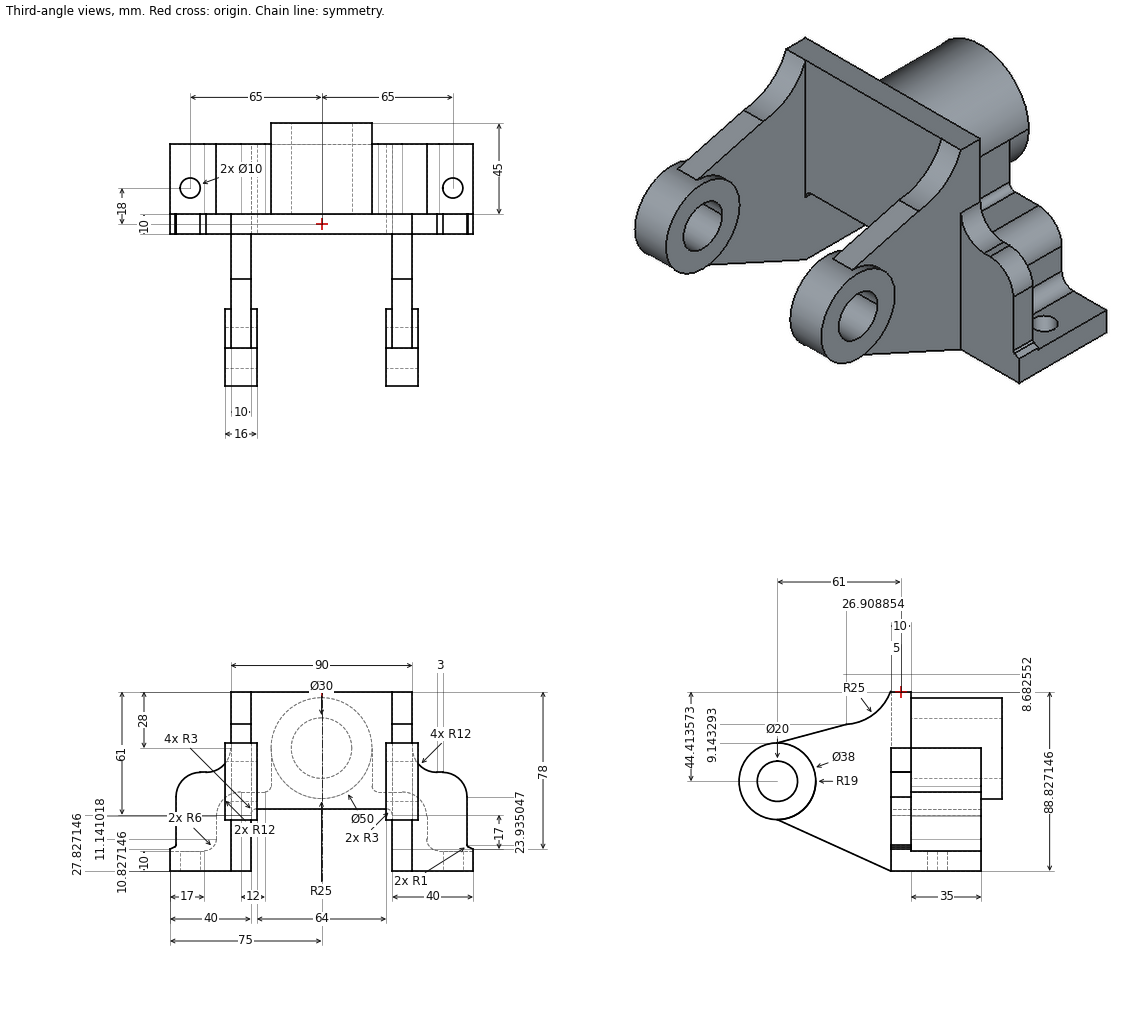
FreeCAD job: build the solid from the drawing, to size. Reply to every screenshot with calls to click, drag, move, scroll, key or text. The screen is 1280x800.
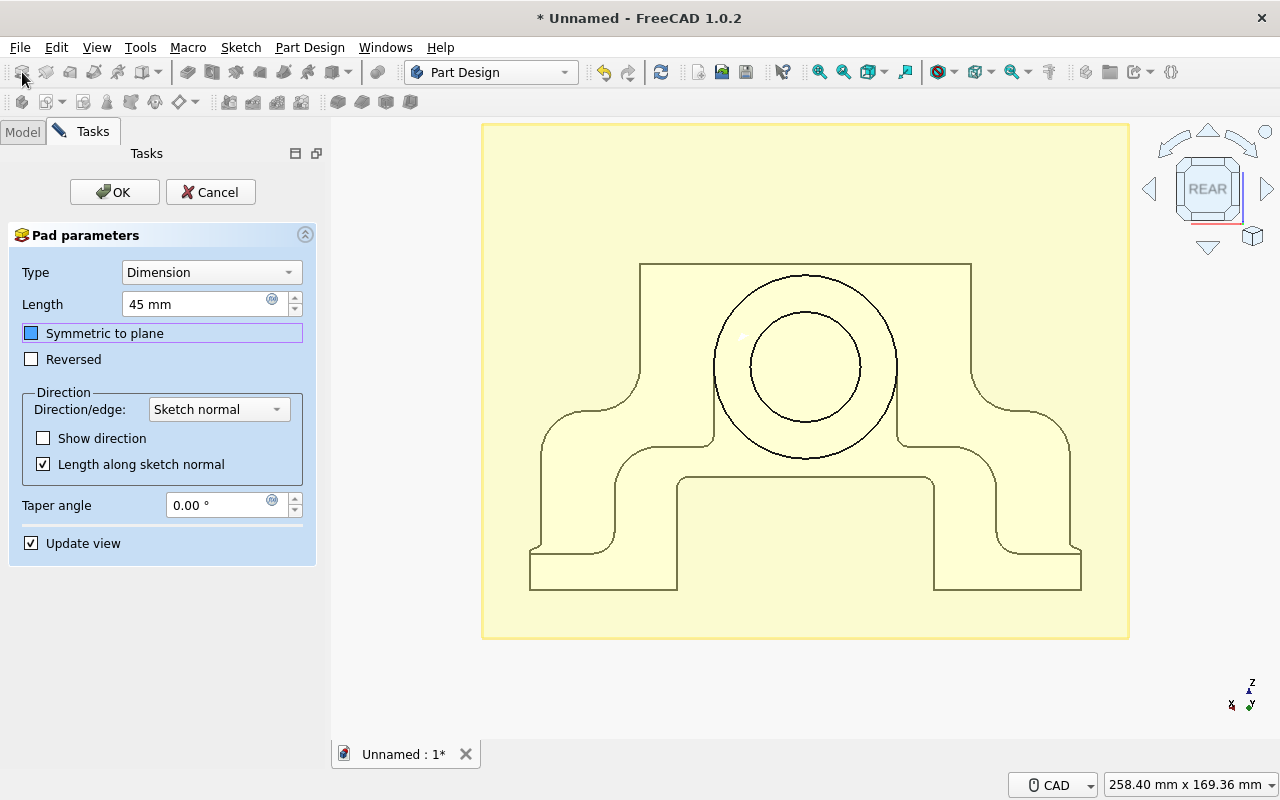
click(115, 192)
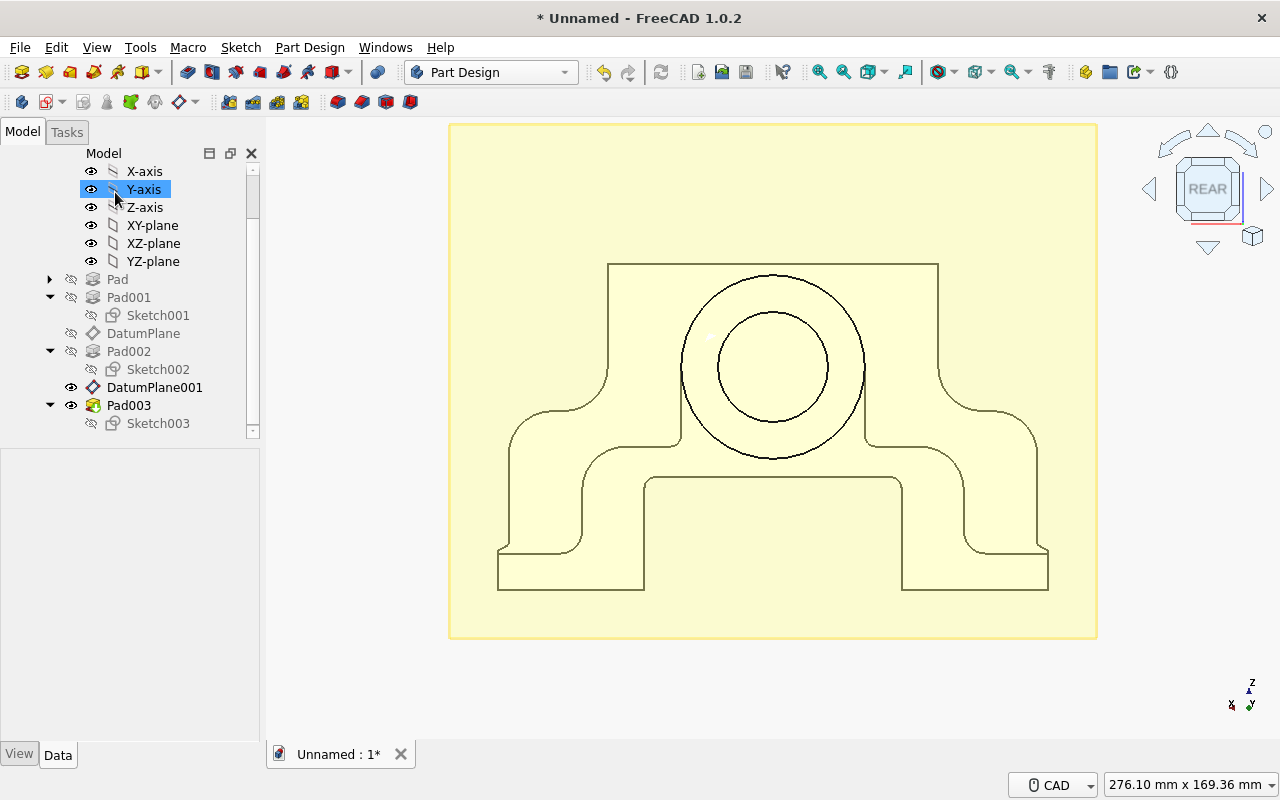
click(116, 387)
key(space)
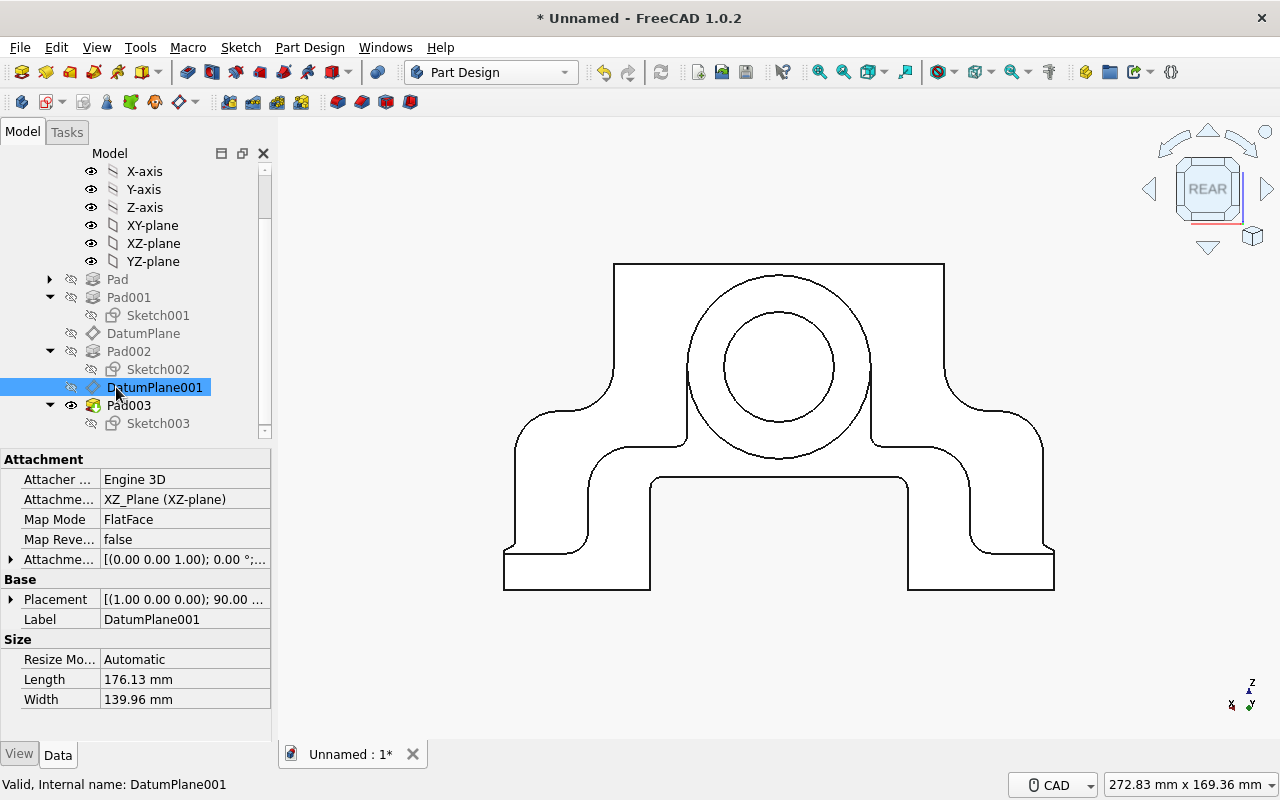
key(5)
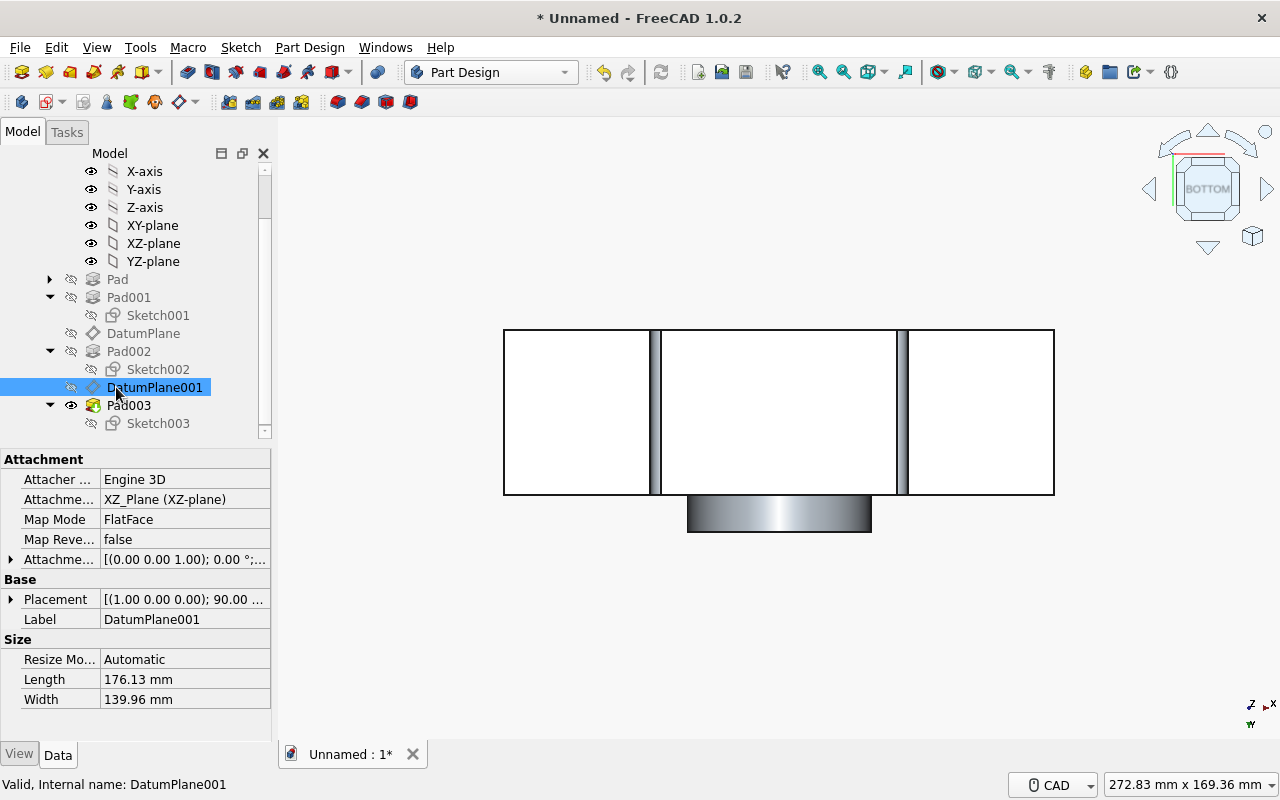
click(577, 411)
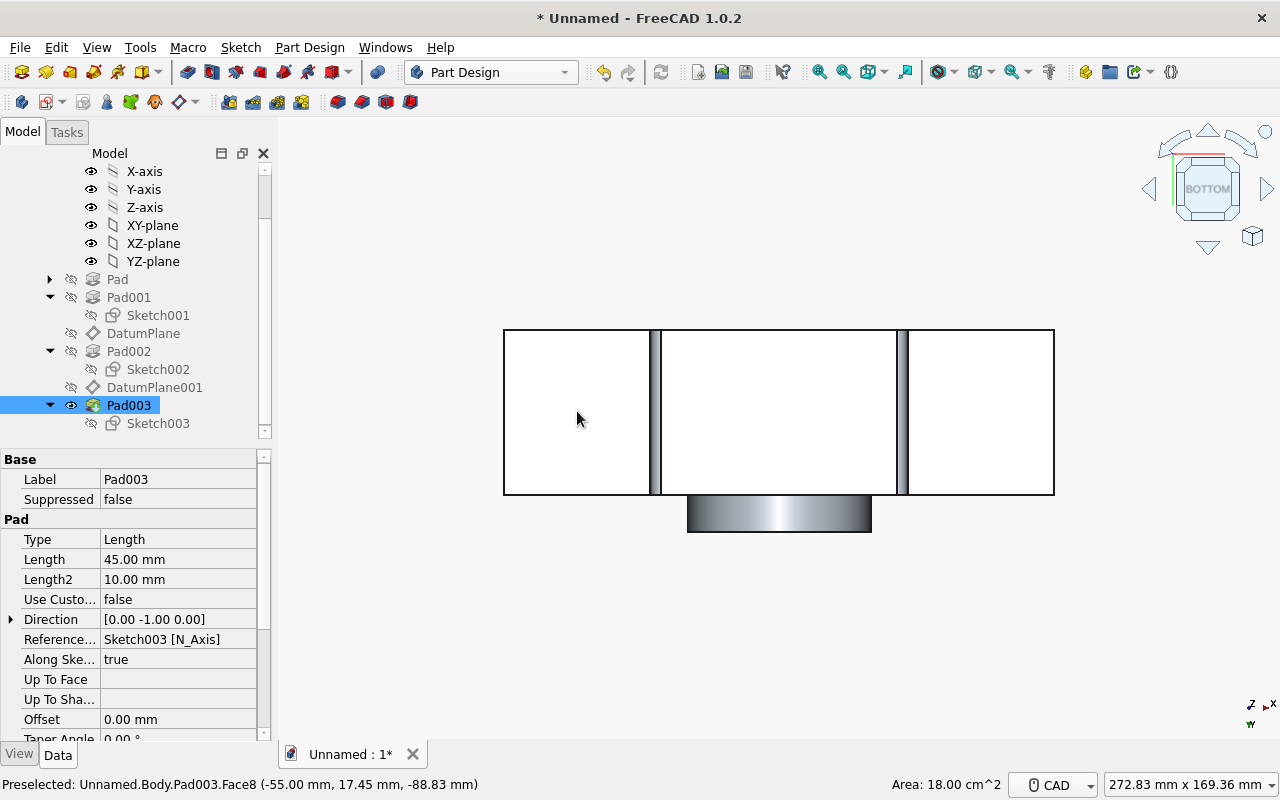
click(46, 102)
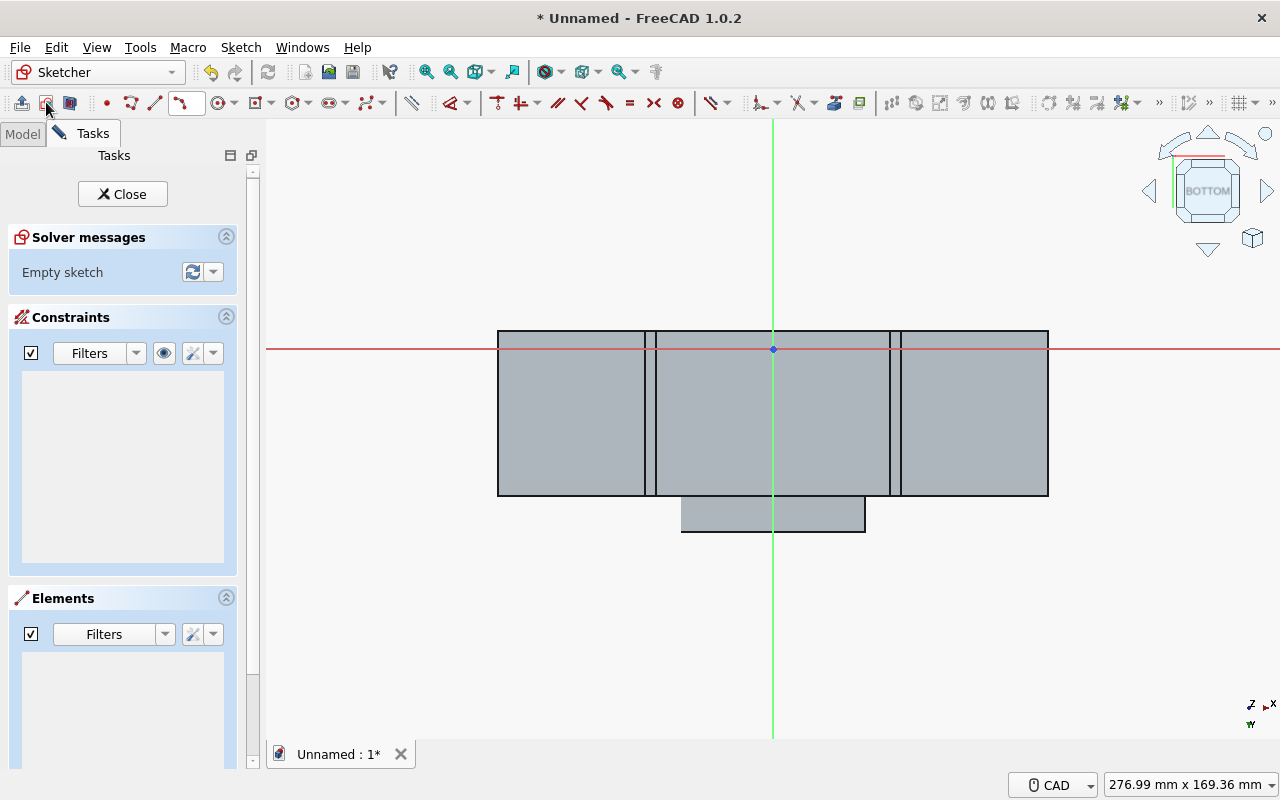
key(g)
key(c)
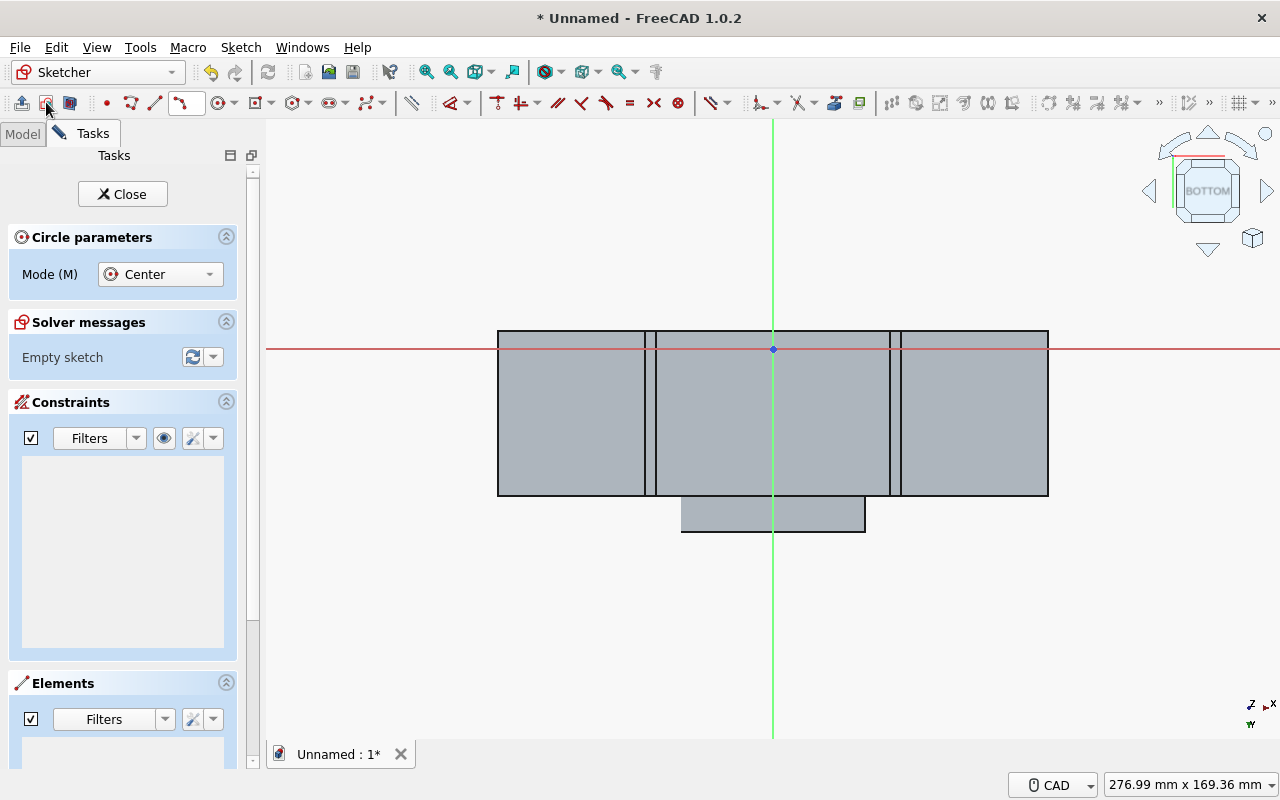
scroll(535, 415, up, 2)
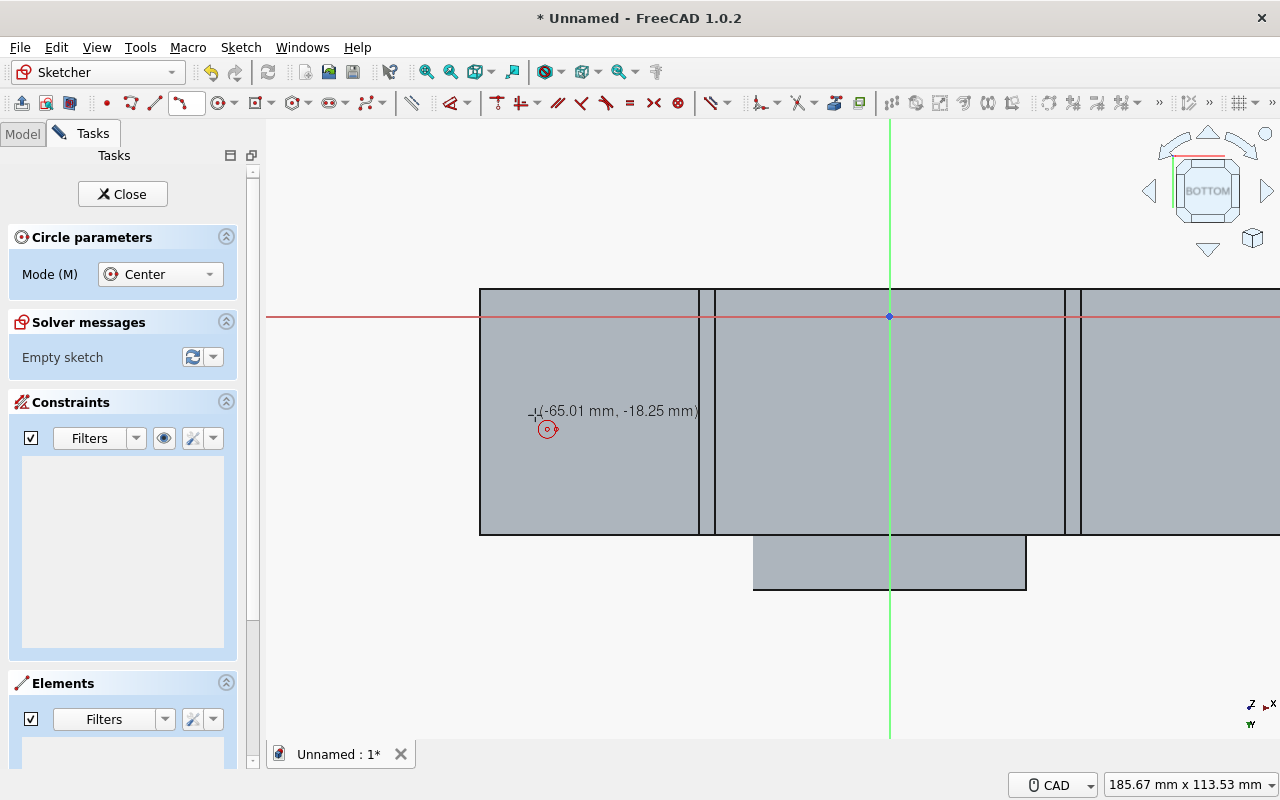
click(535, 415)
click(554, 396)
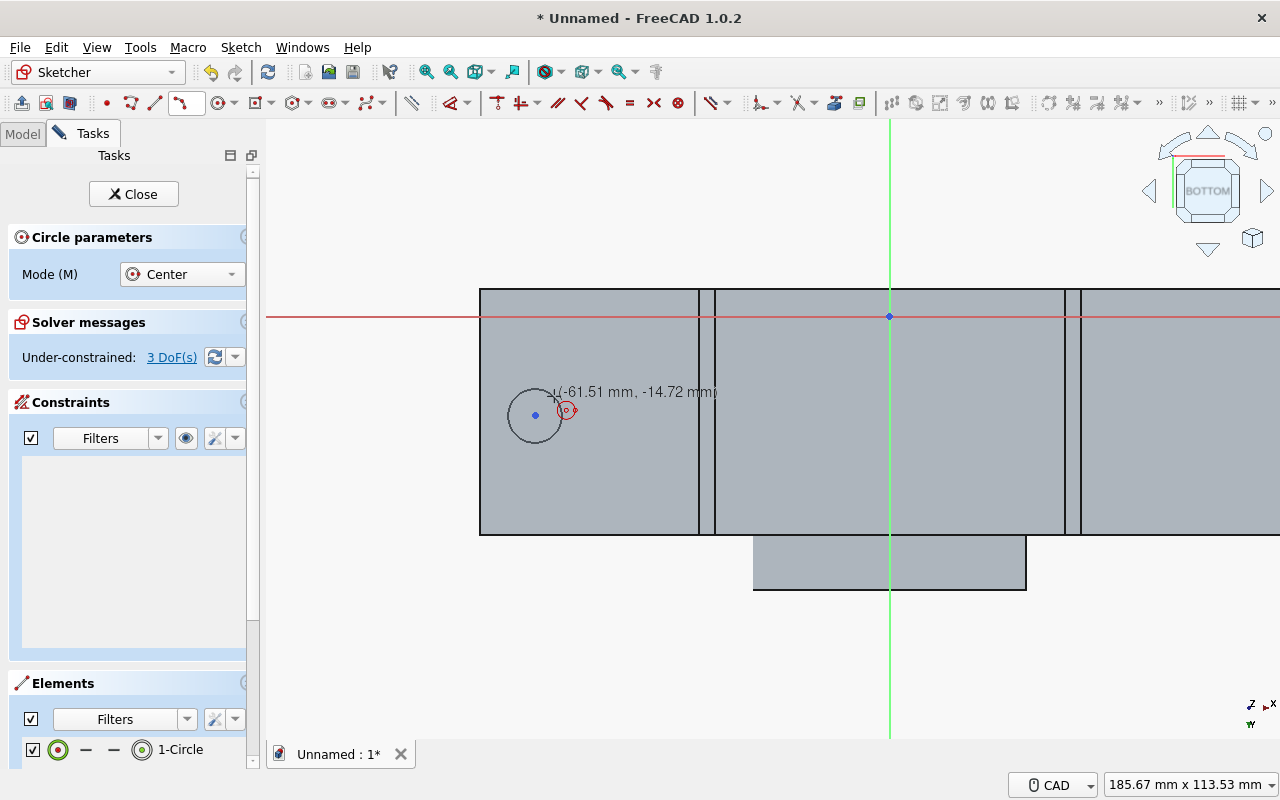
scroll(327, 530, down, 2)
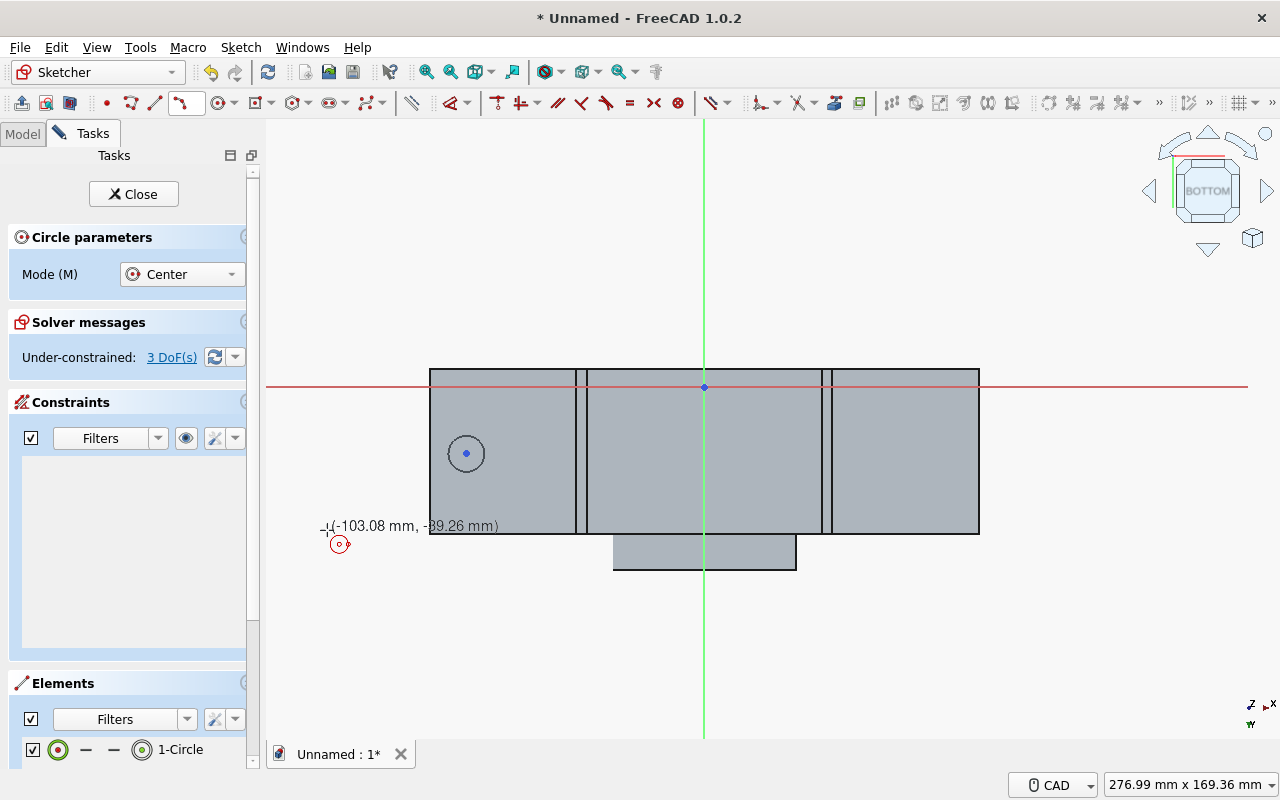
scroll(942, 453, up, 2)